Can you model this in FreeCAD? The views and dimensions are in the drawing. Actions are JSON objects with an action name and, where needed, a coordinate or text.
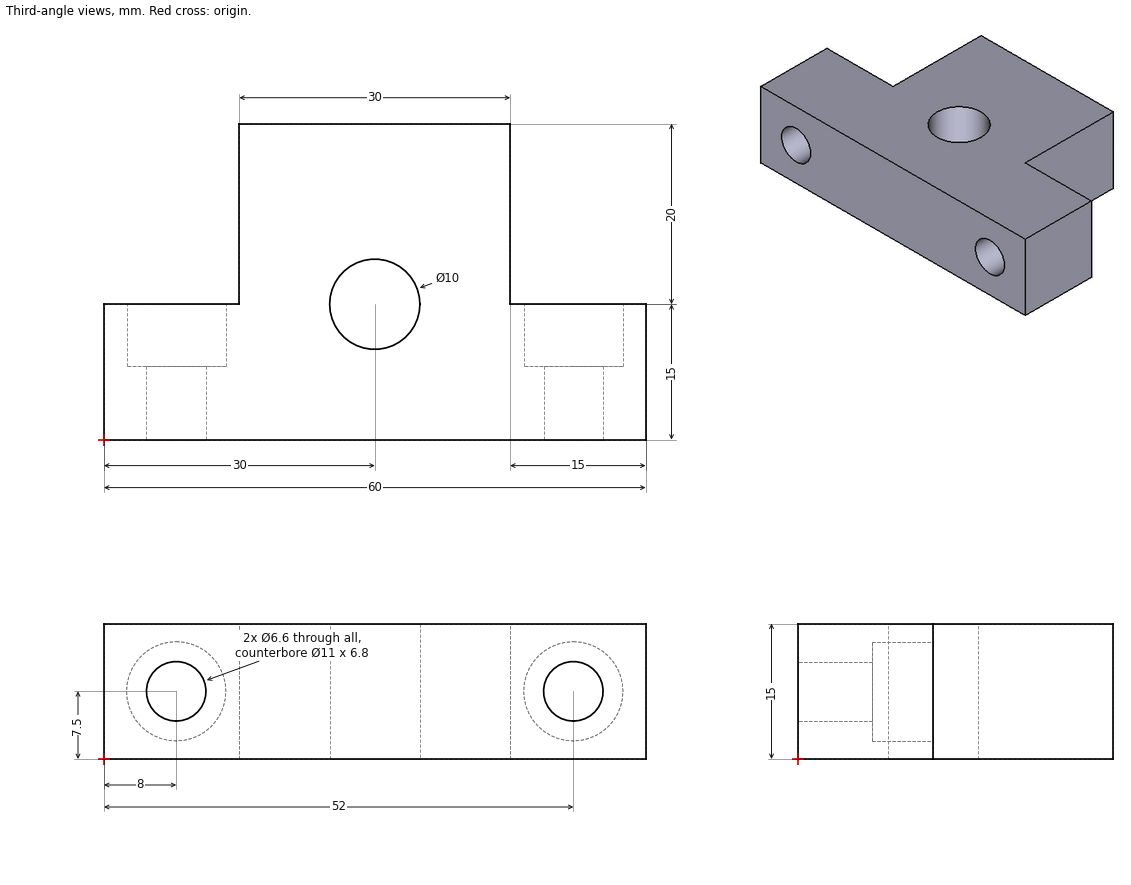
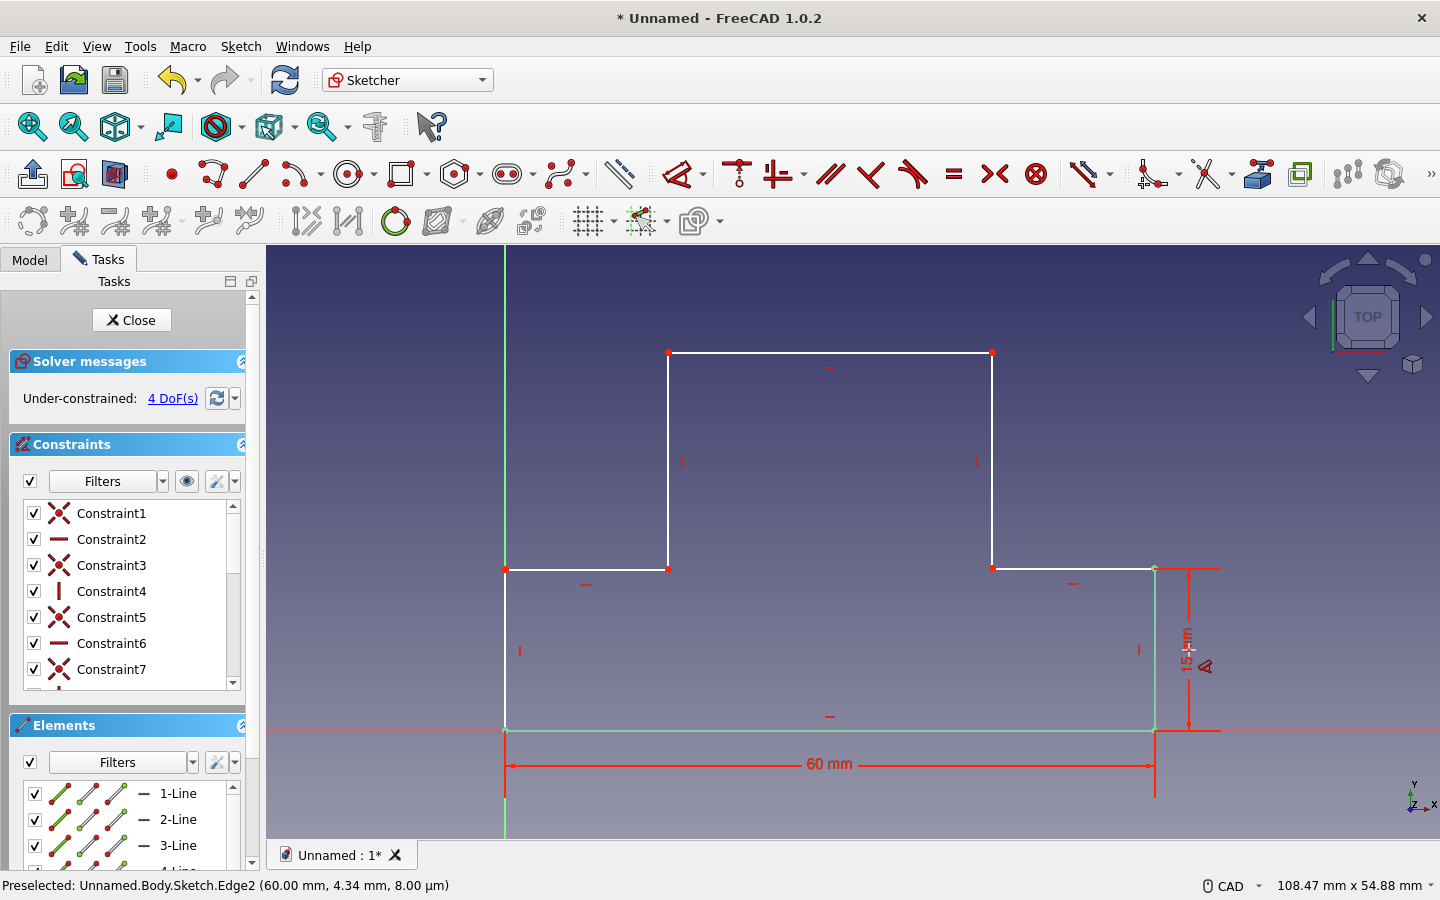
{"action": "left_click", "coordinate": [1106, 569]}
{"action": "left_click", "coordinate": [1073, 603]}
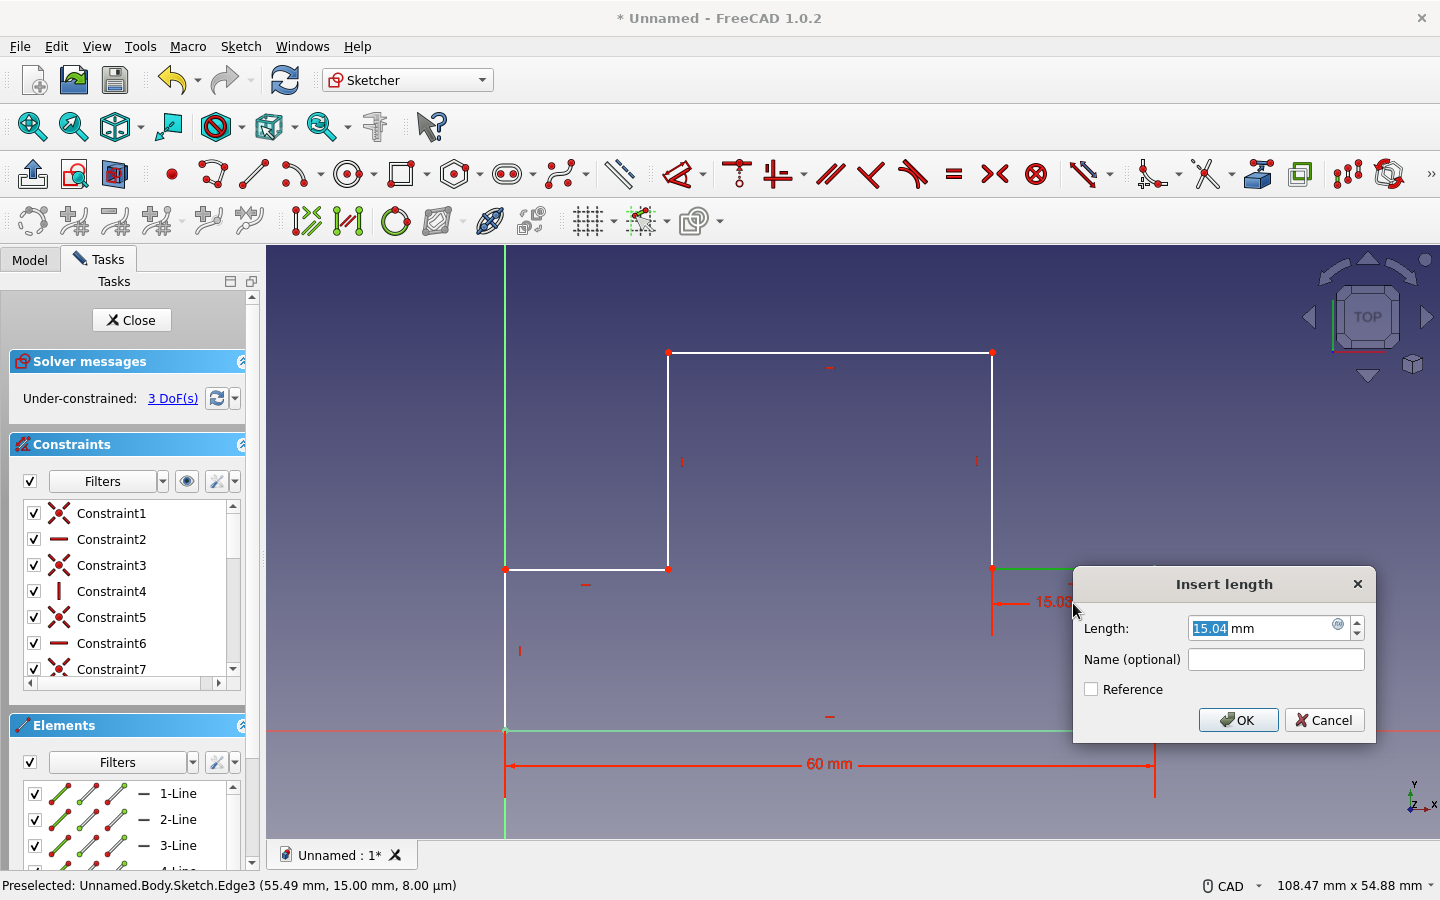
{"action": "type", "text": "15"}
{"action": "key", "text": "Return"}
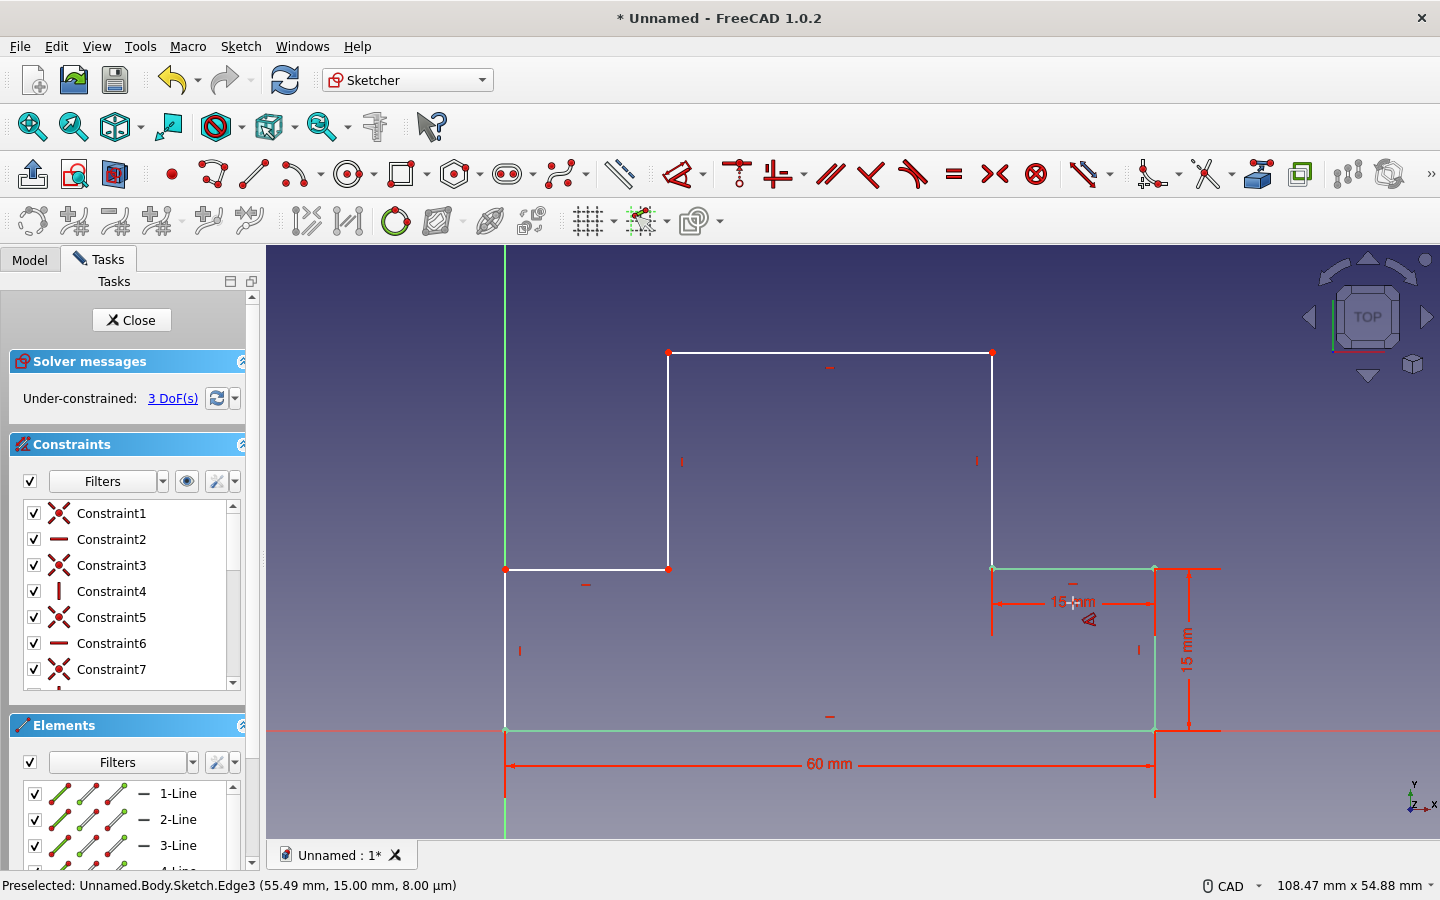
{"action": "left_click", "coordinate": [992, 504]}
{"action": "left_click", "coordinate": [1026, 461]}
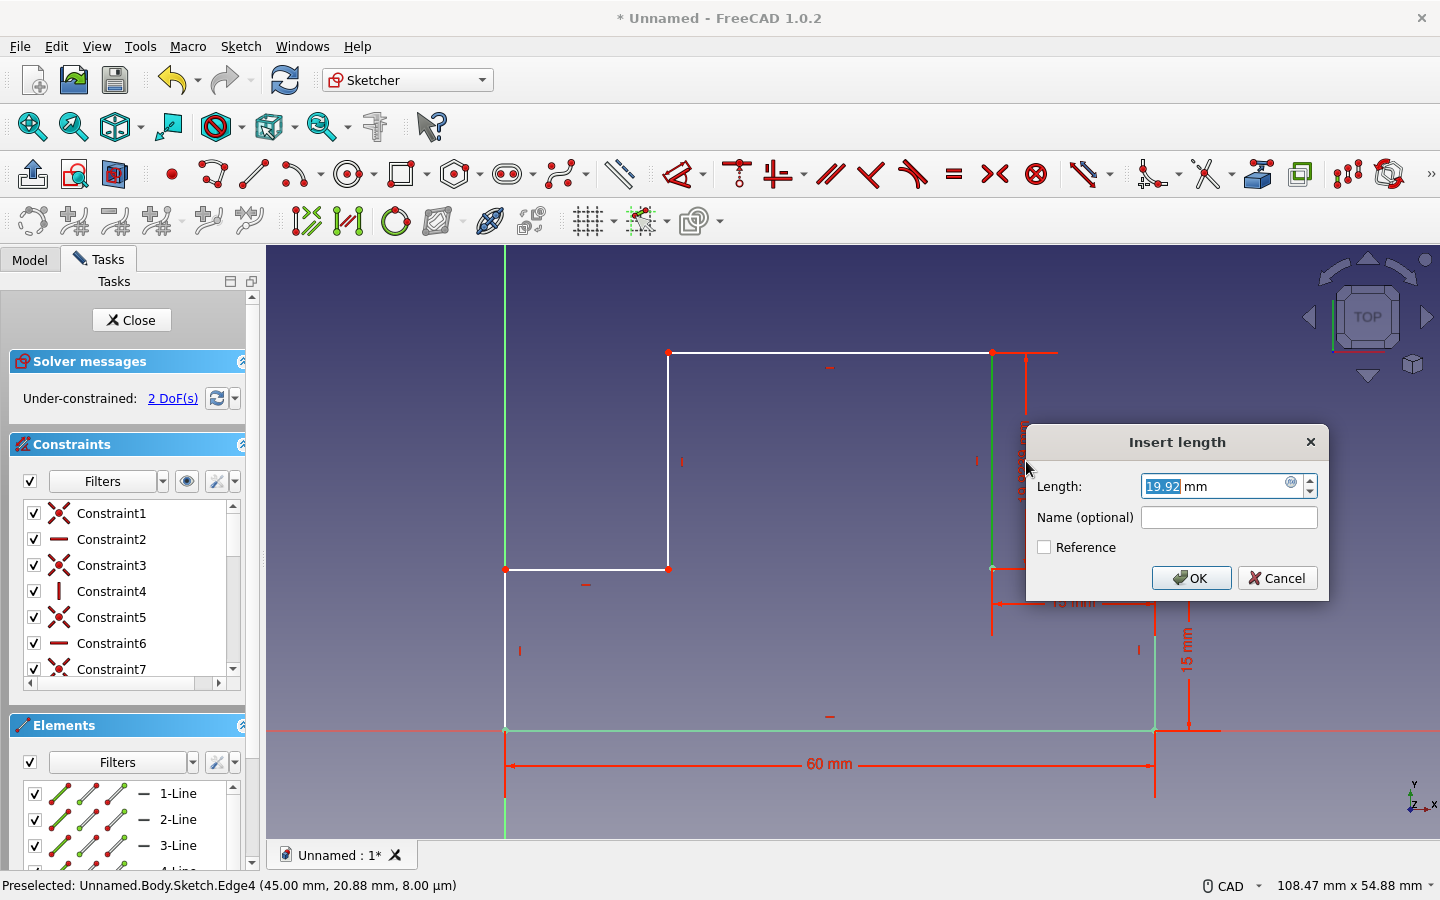
{"action": "type", "text": "20"}
{"action": "key", "text": "Return"}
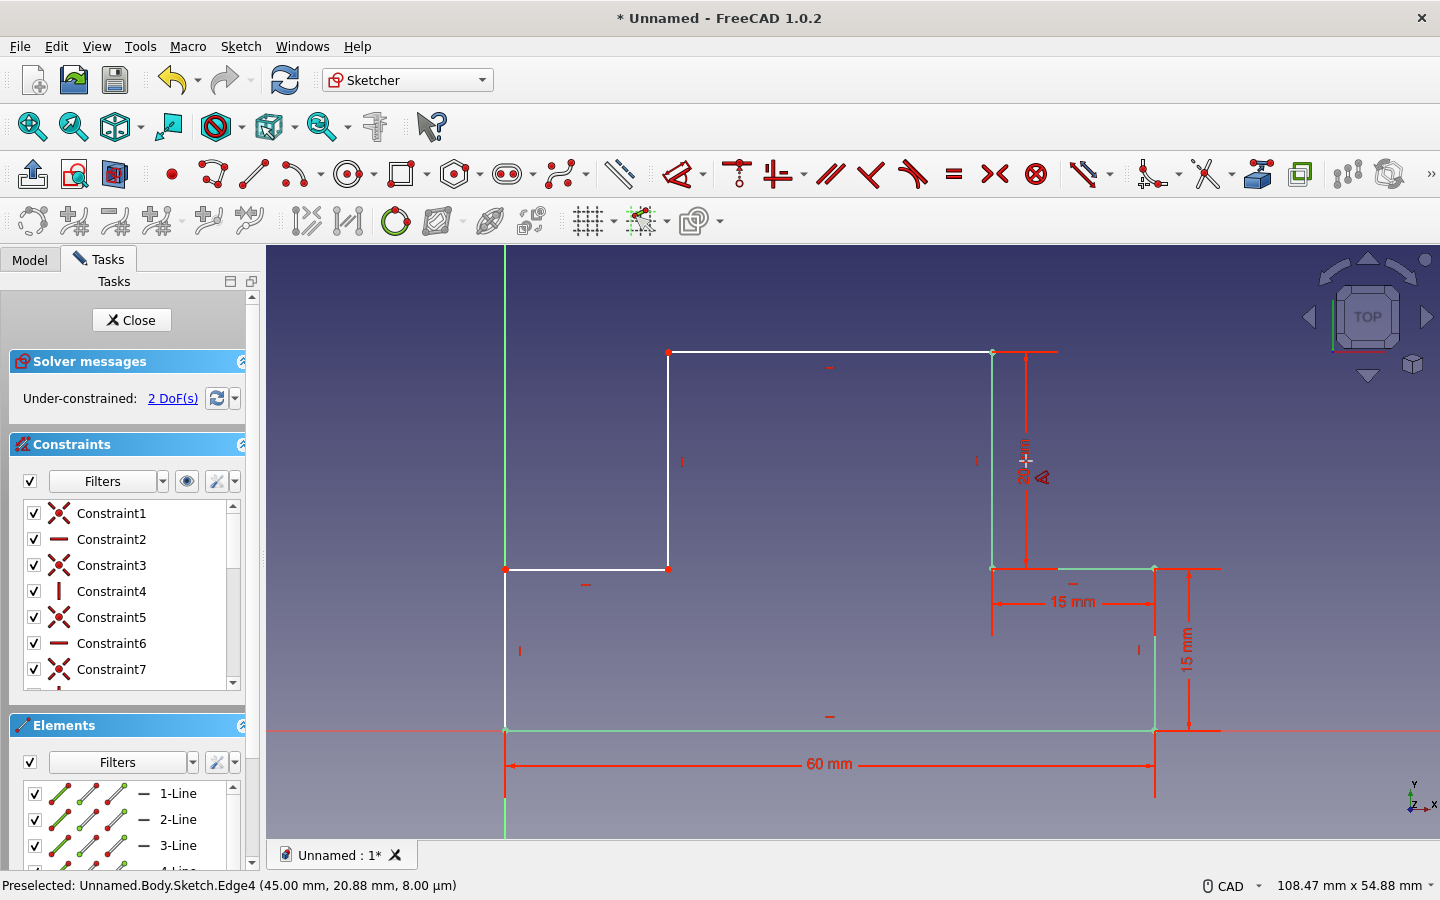
{"action": "left_click", "coordinate": [895, 352]}
{"action": "left_click", "coordinate": [830, 318]}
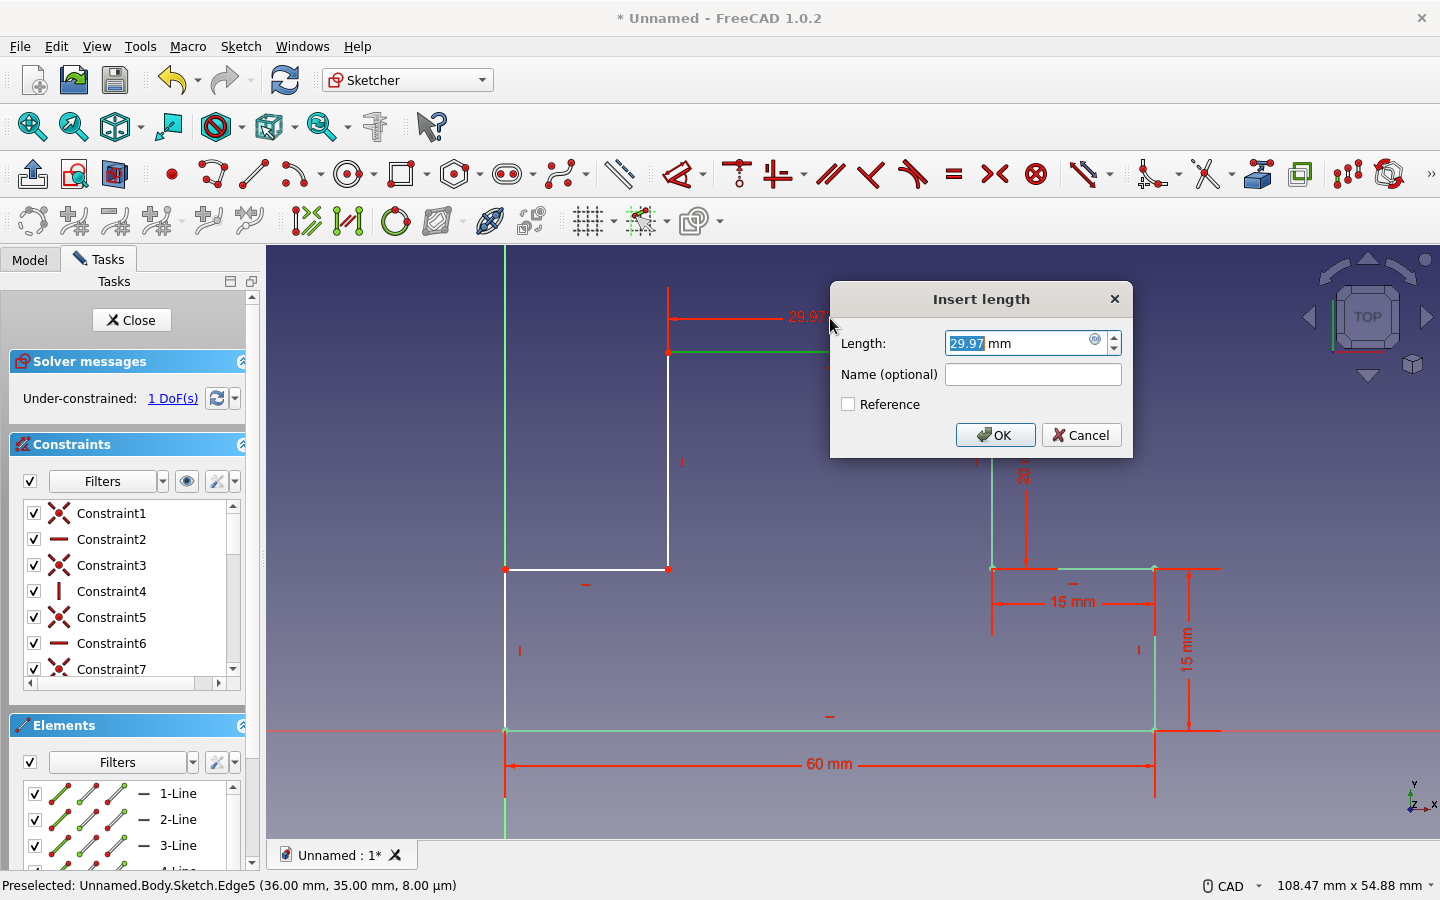
{"action": "type", "text": "30"}
{"action": "key", "text": "Return"}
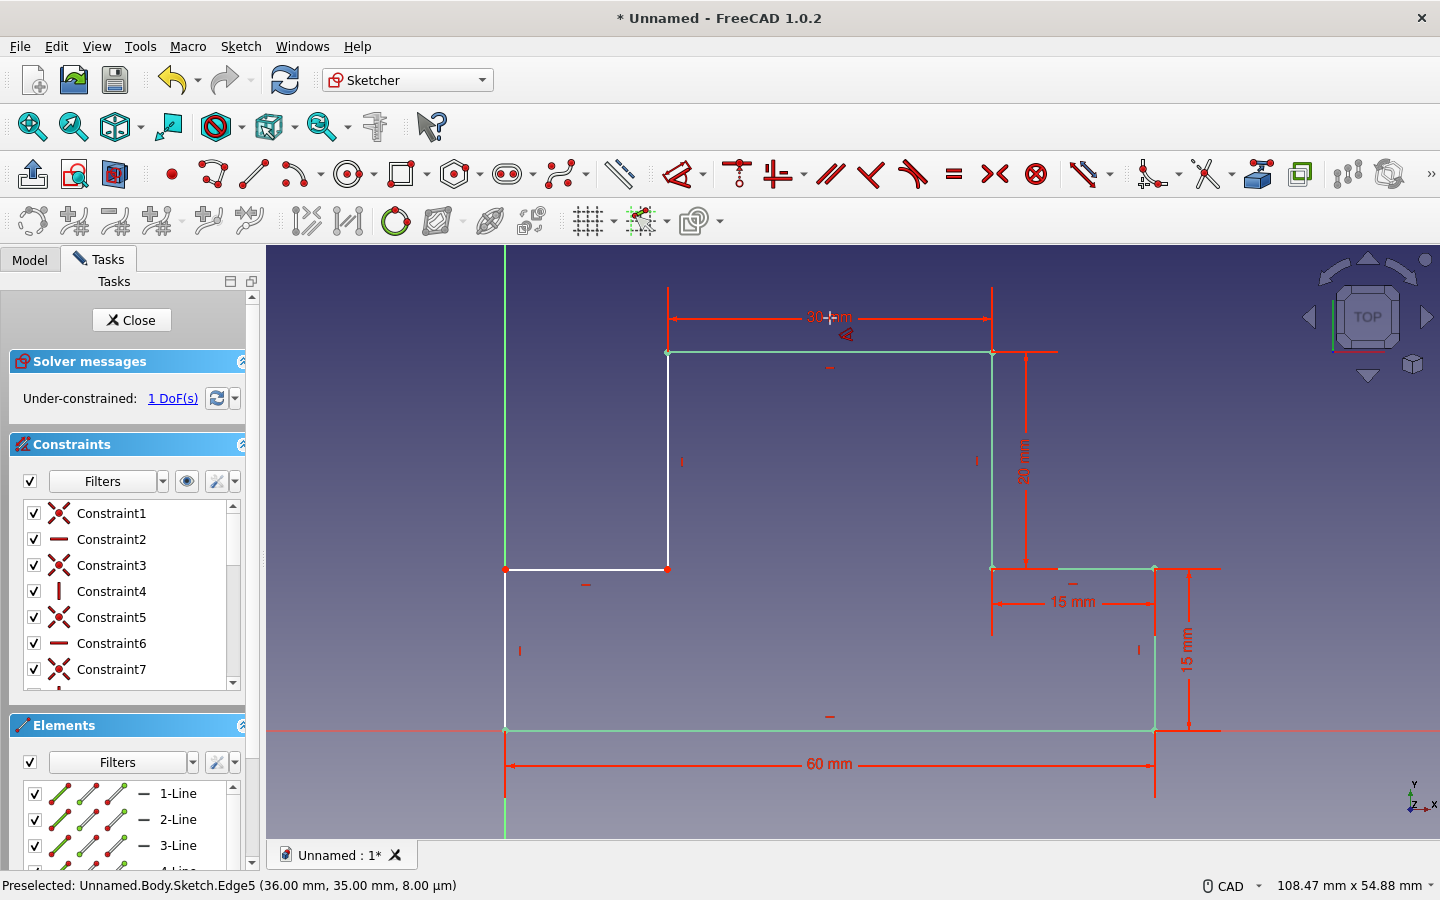
{"action": "left_click", "coordinate": [668, 418]}
{"action": "left_click", "coordinate": [634, 461]}